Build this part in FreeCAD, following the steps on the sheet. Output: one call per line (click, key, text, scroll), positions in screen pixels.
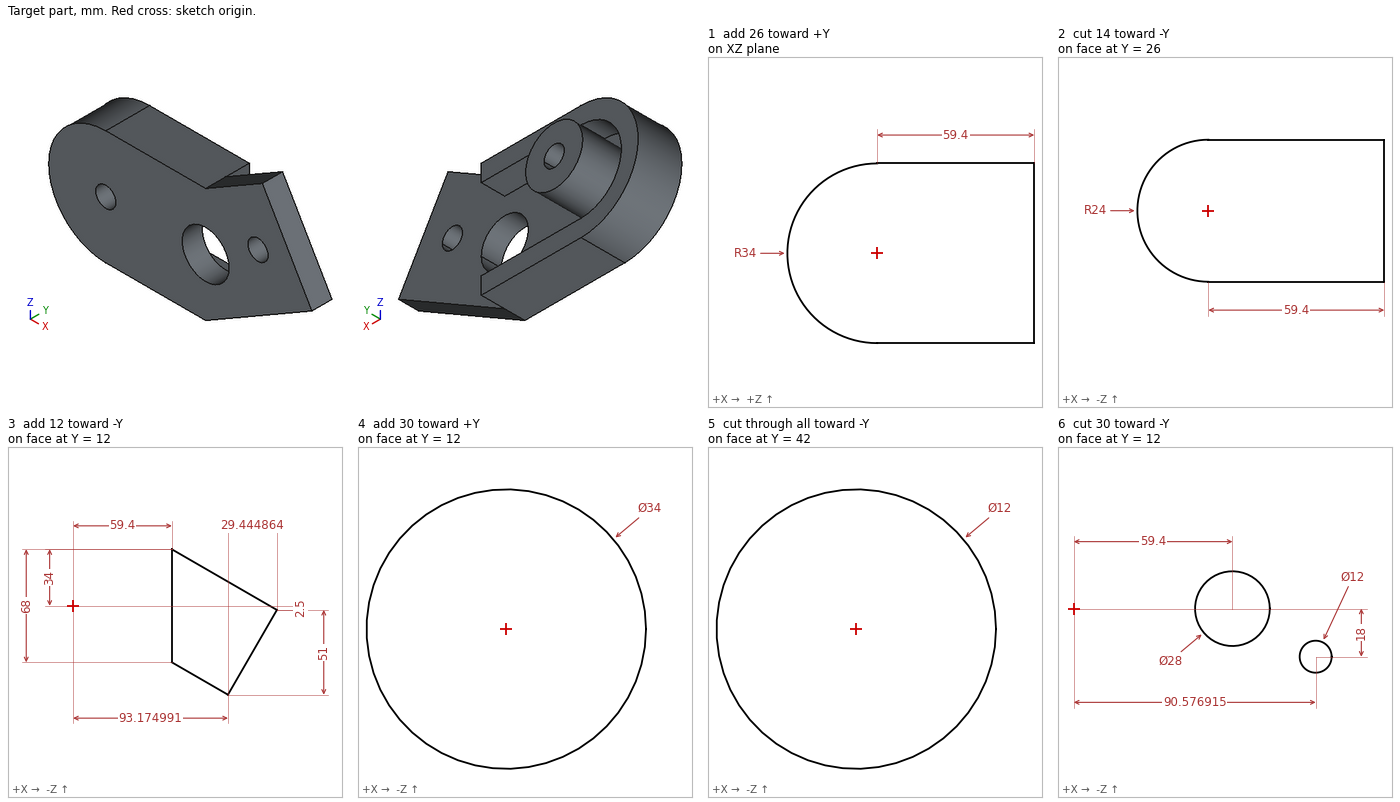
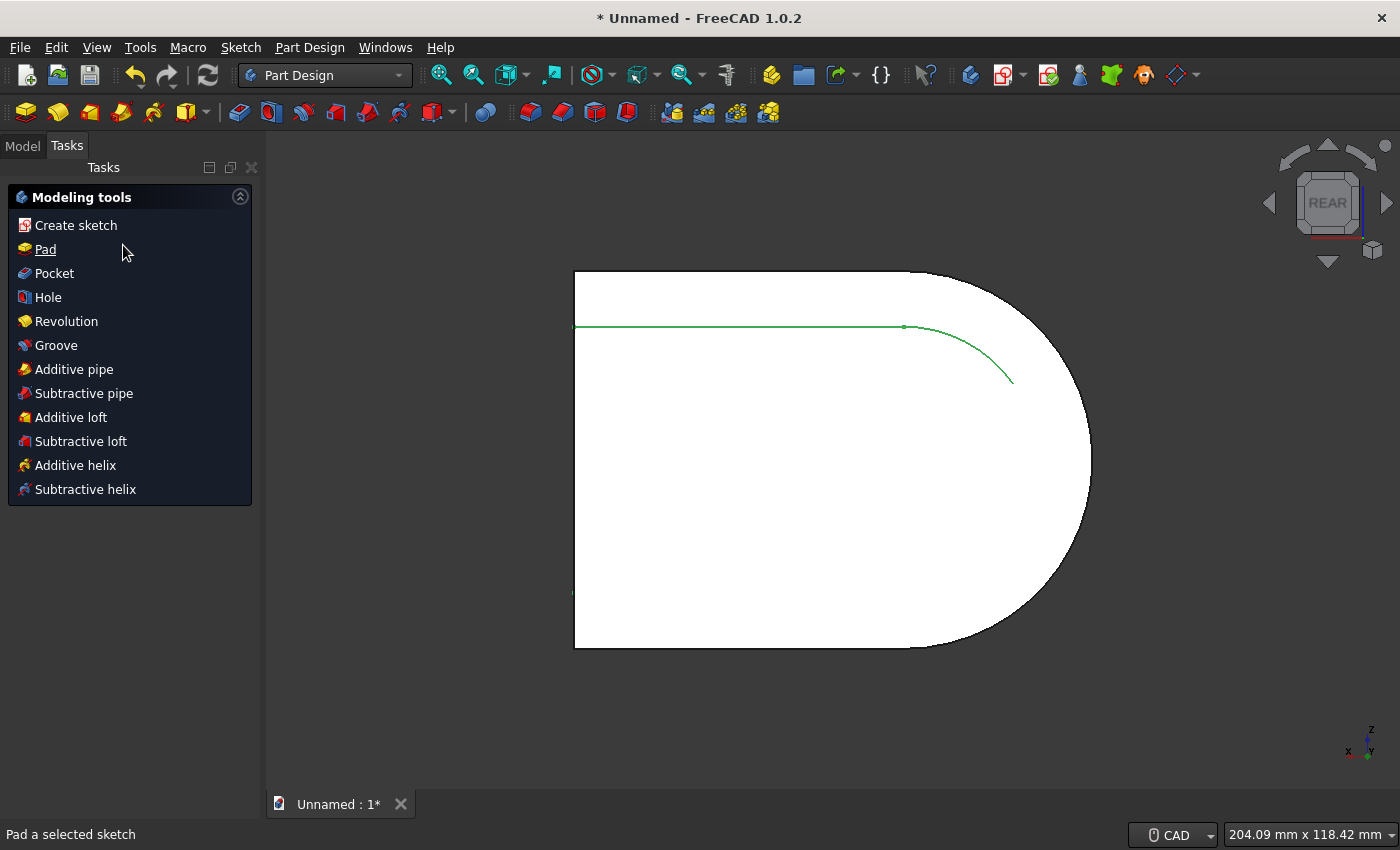
click(240, 112)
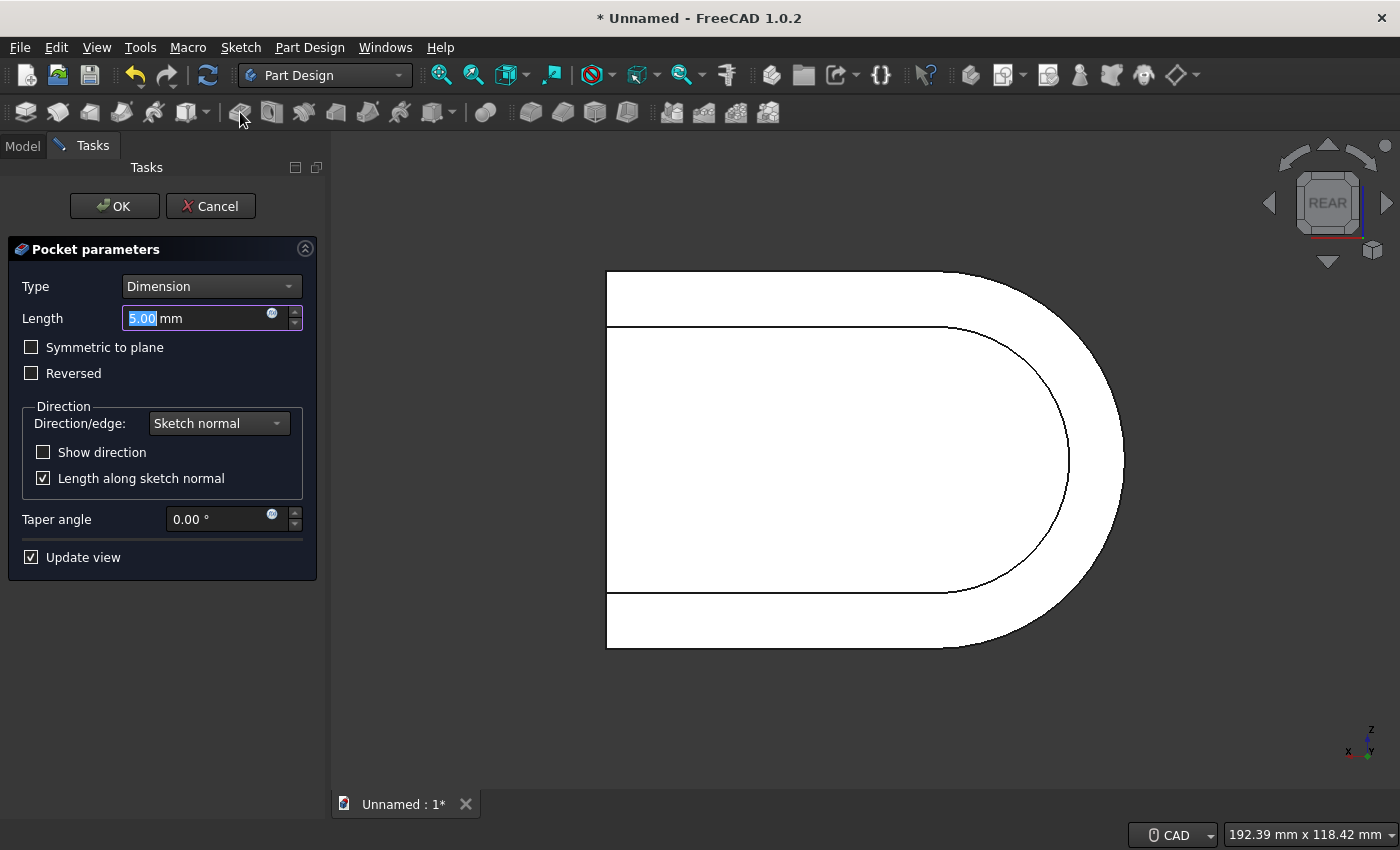
text(14)
key(Tab)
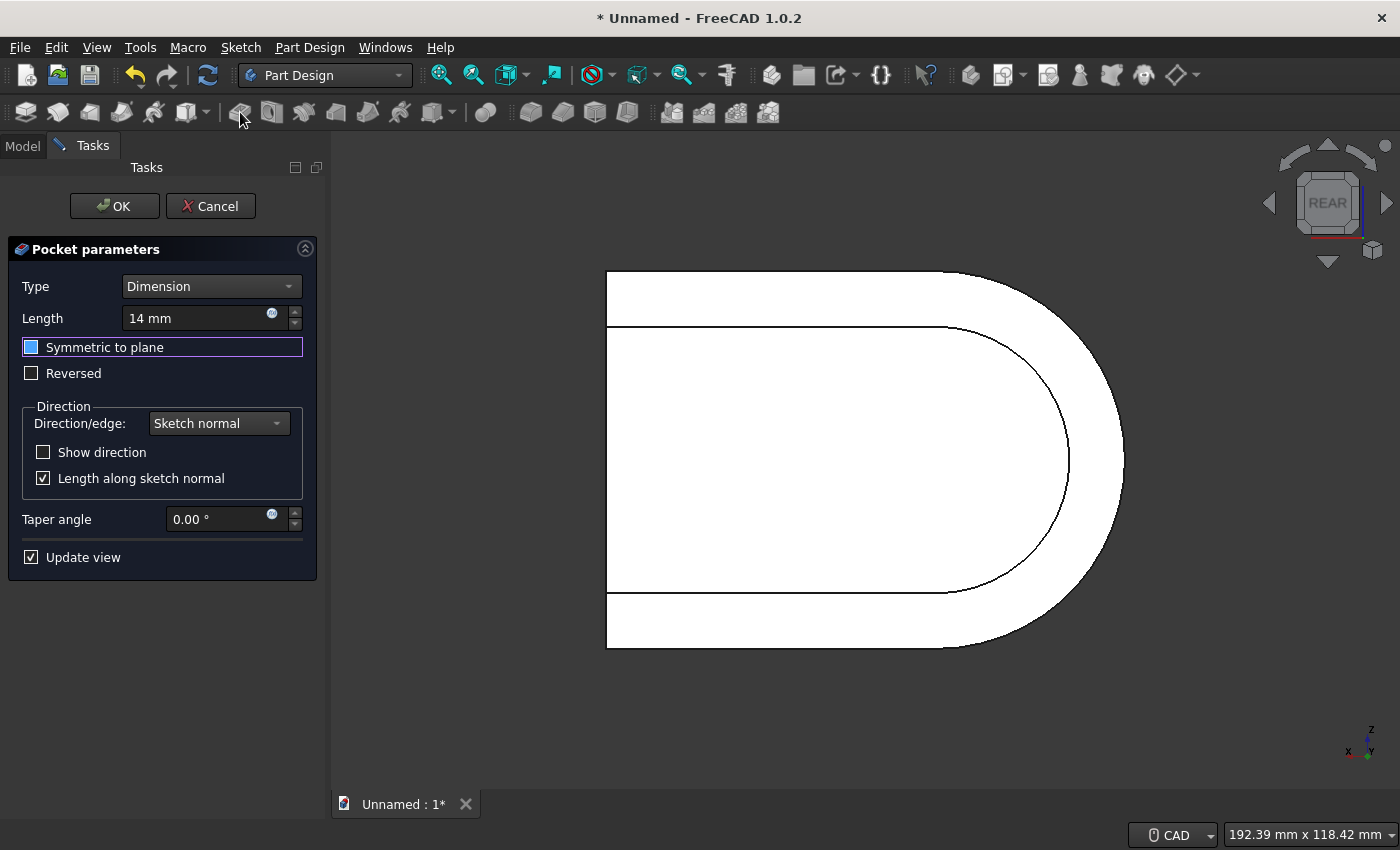
click(115, 206)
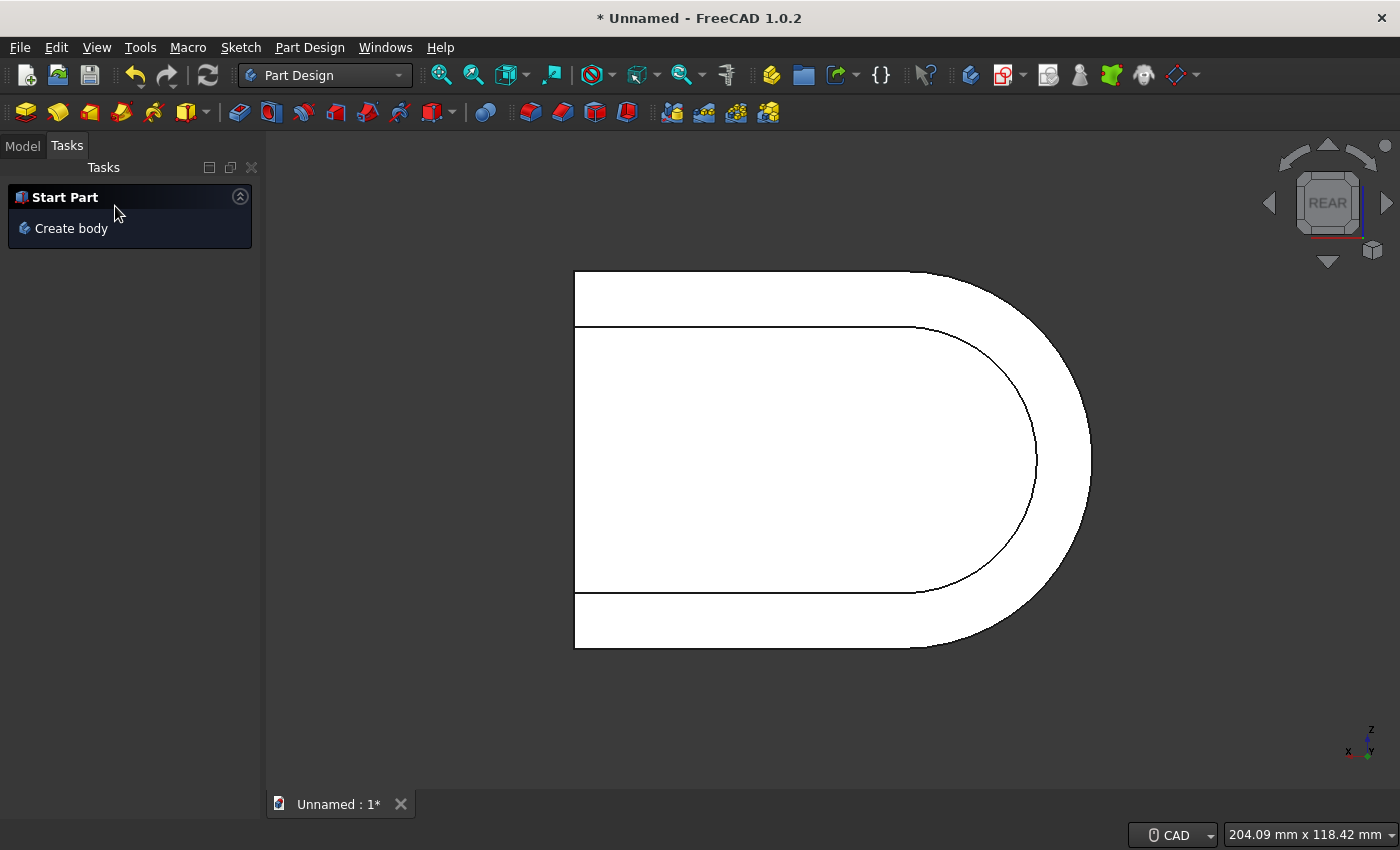
click(739, 459)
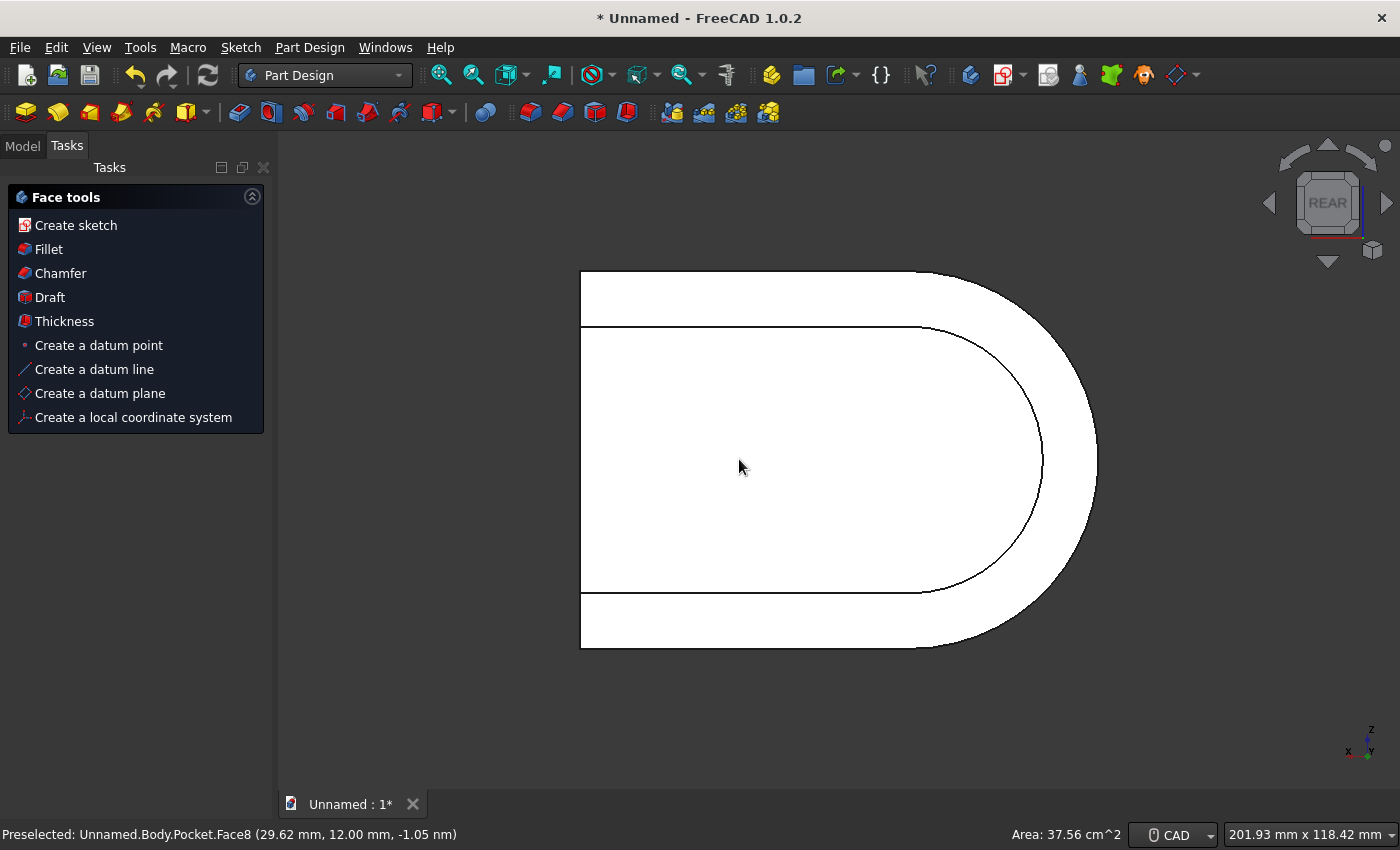
click(1004, 76)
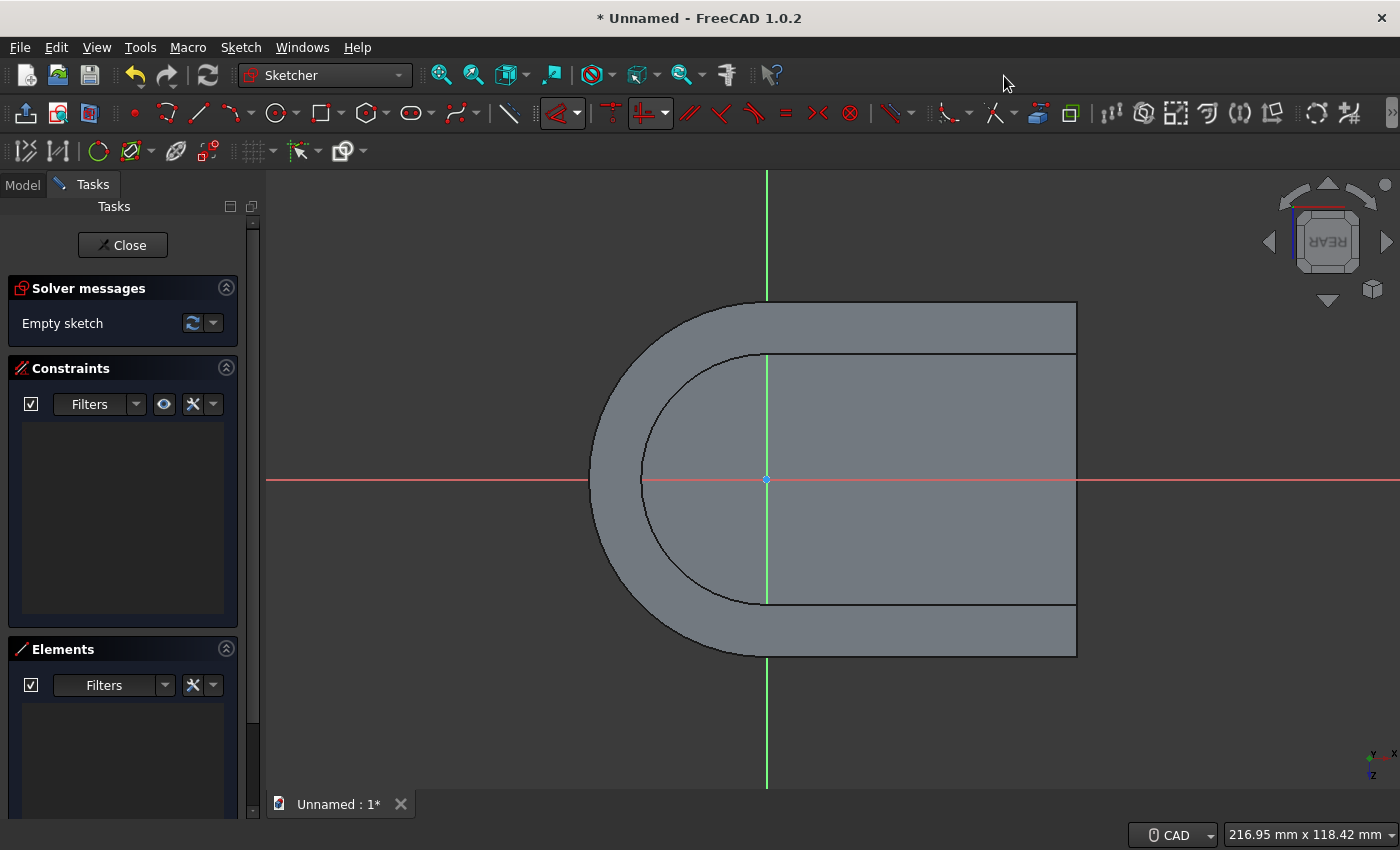
click(90, 114)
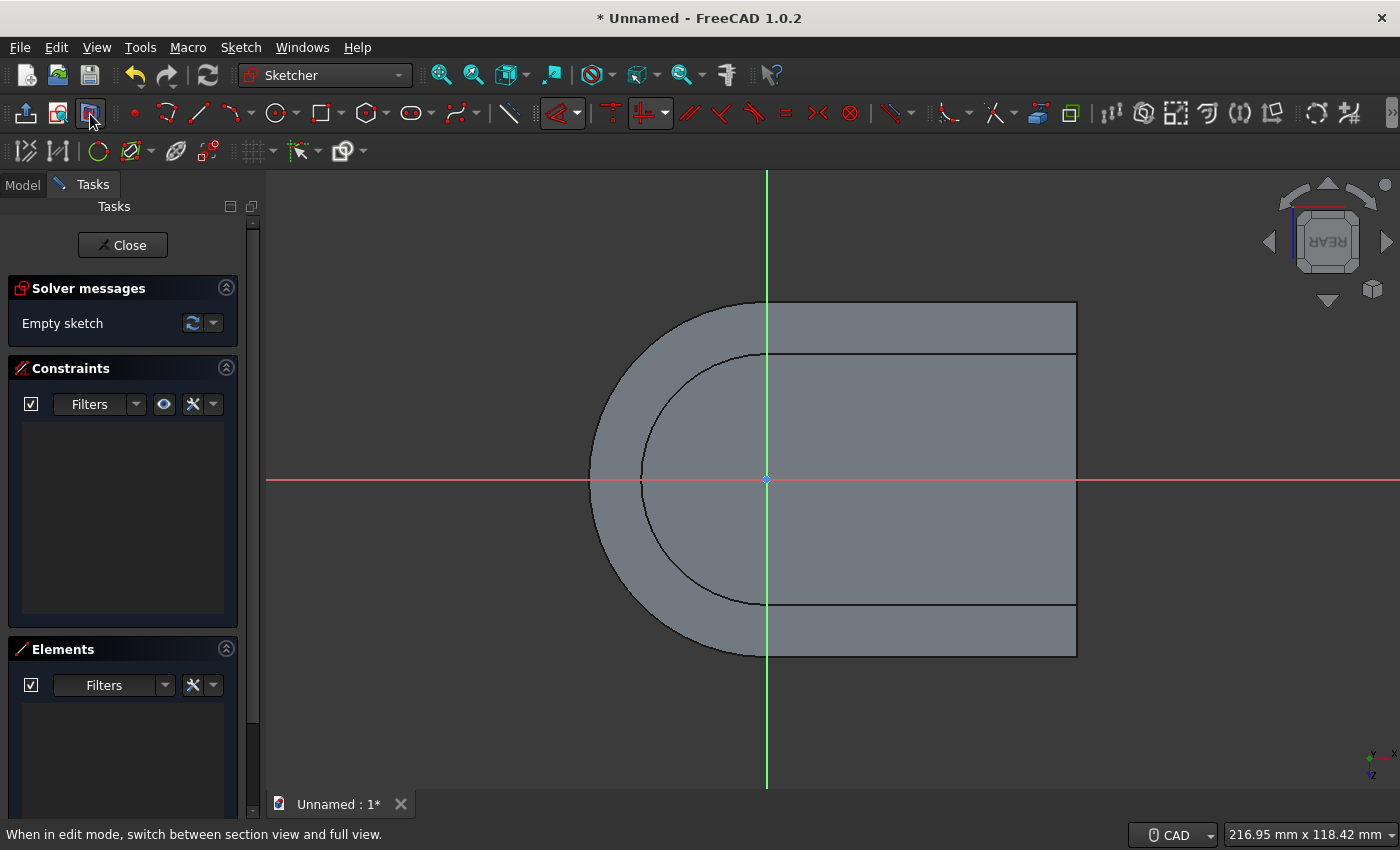
scroll(294, 249, down, 1)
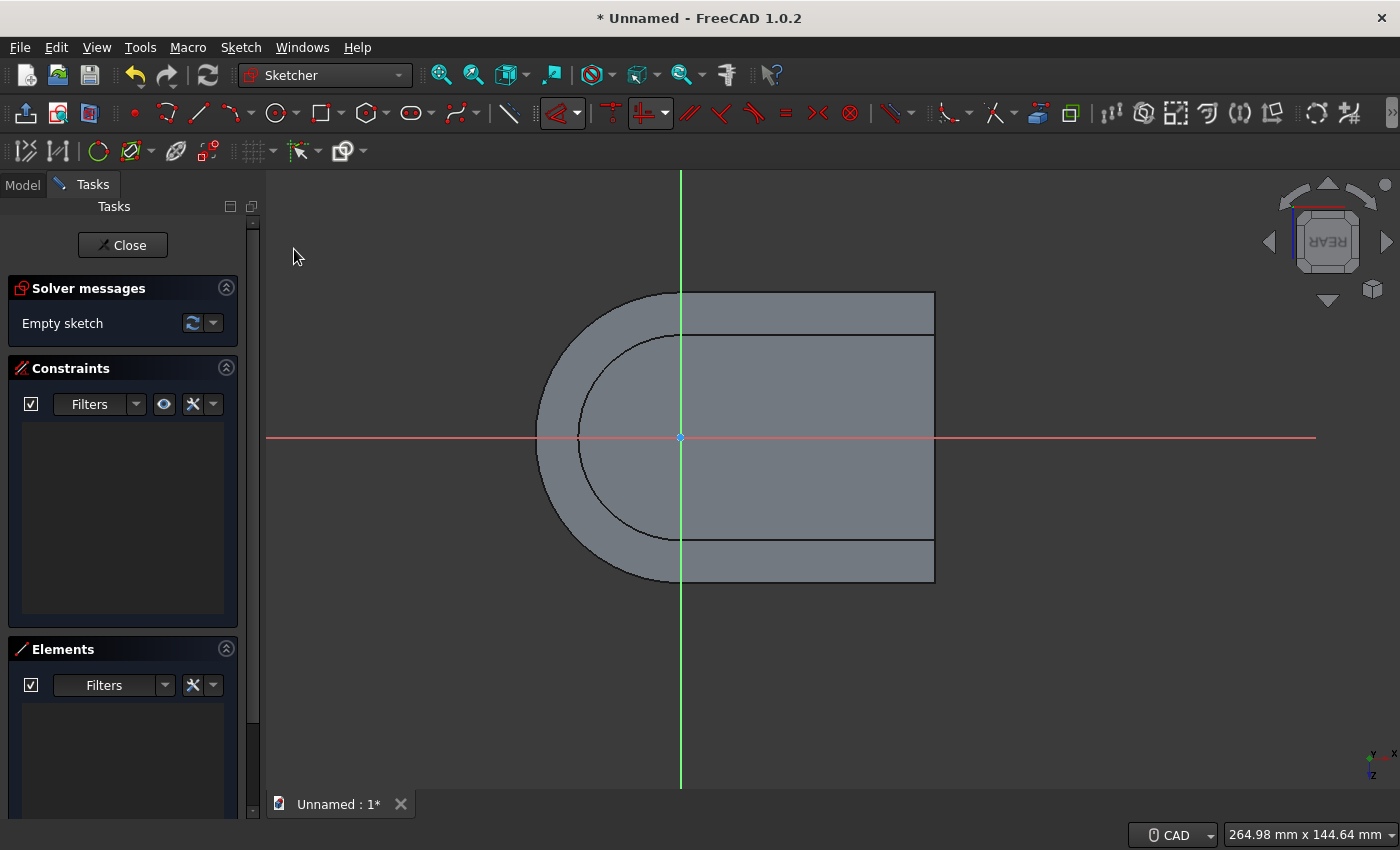
click(168, 114)